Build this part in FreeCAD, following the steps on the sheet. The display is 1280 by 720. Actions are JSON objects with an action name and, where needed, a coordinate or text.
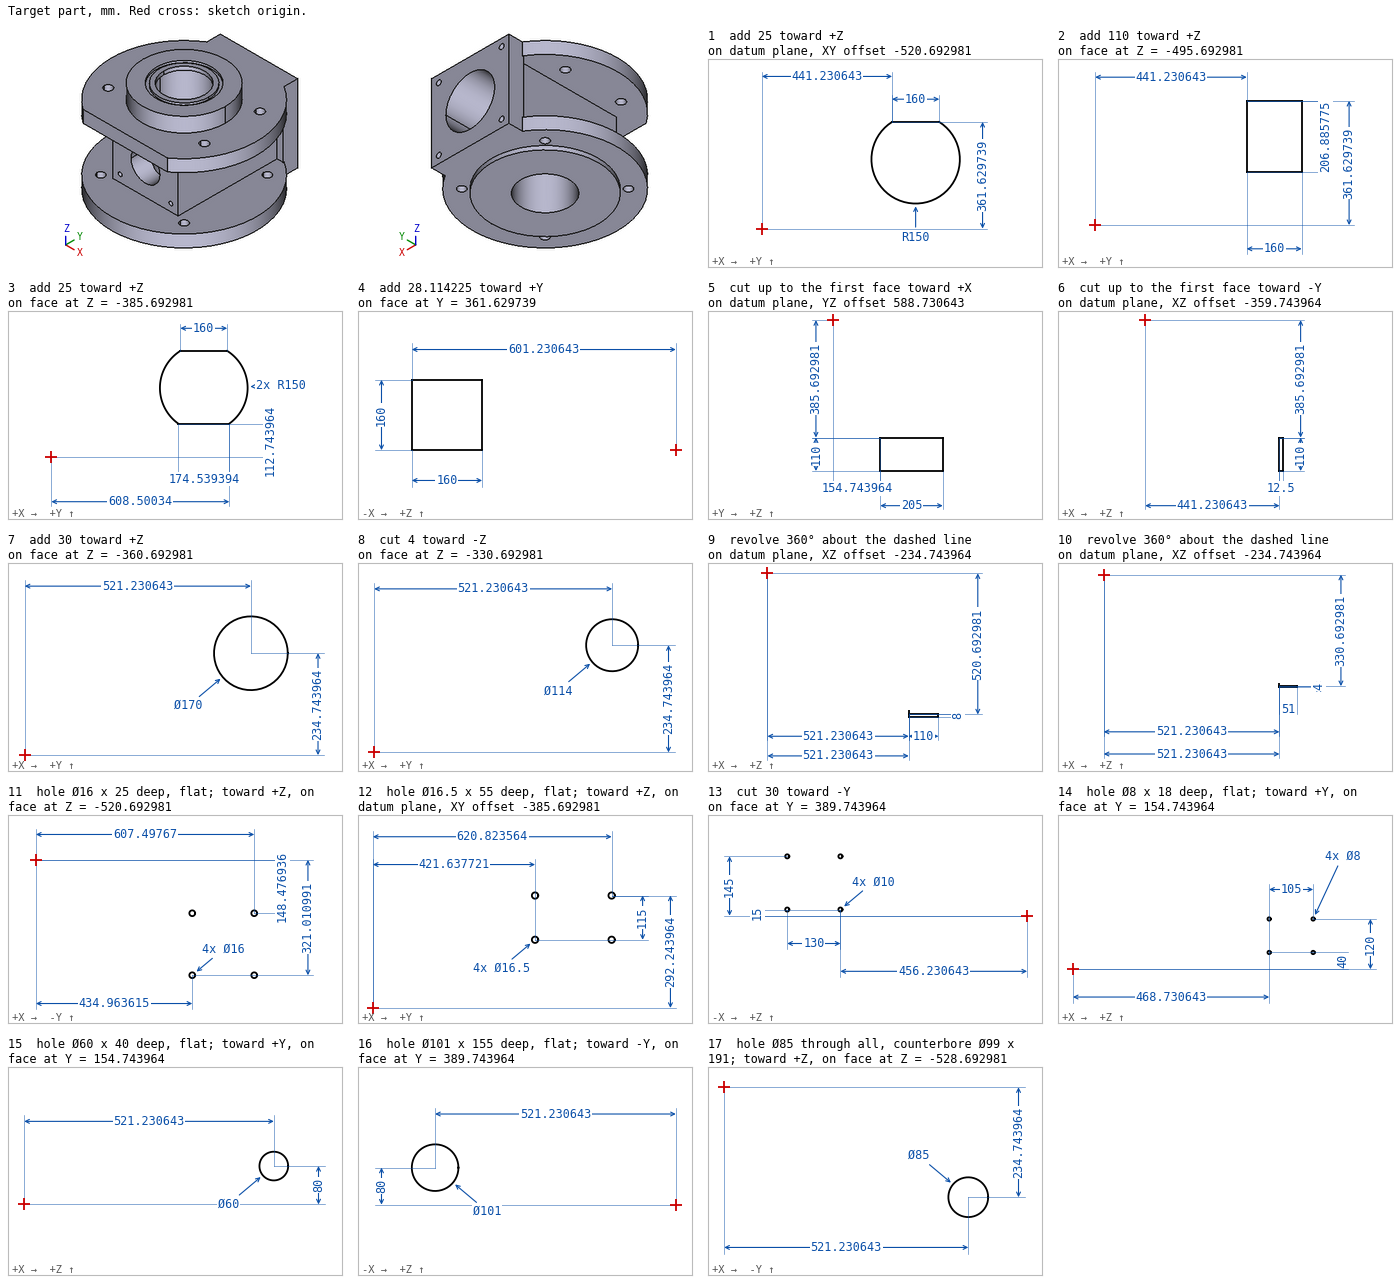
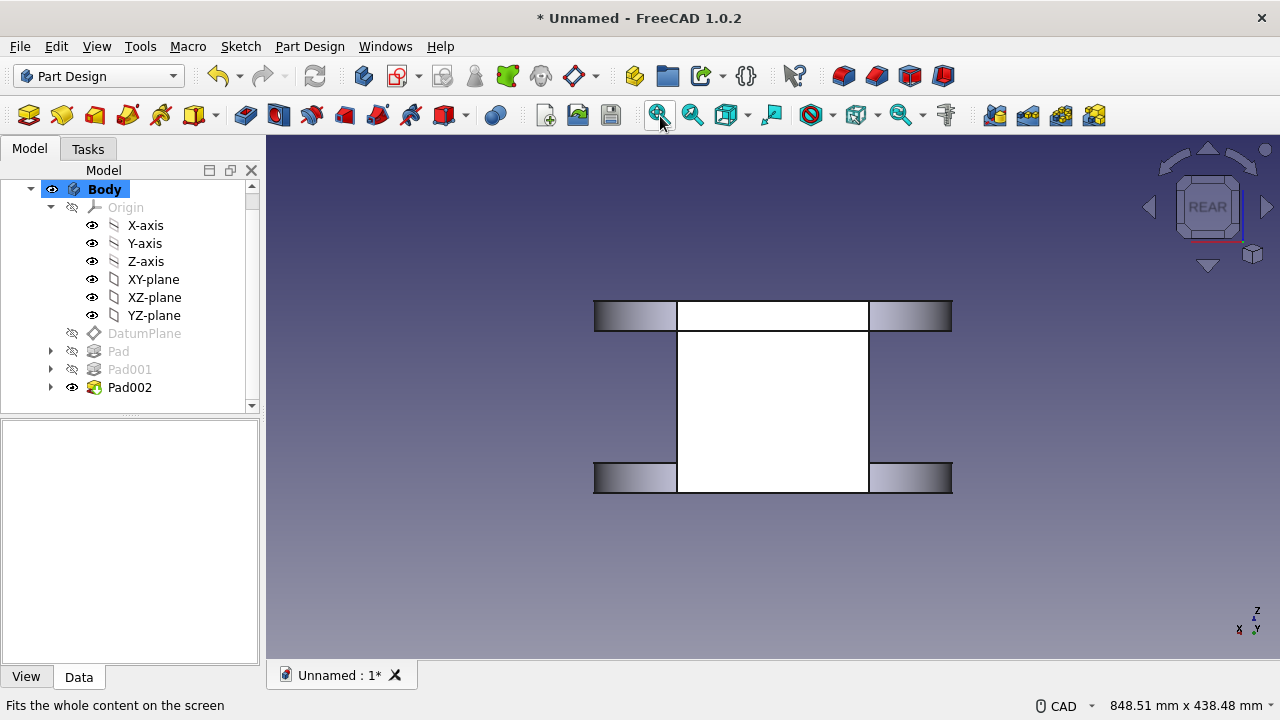
{"action": "left_click", "coordinate": [773, 411]}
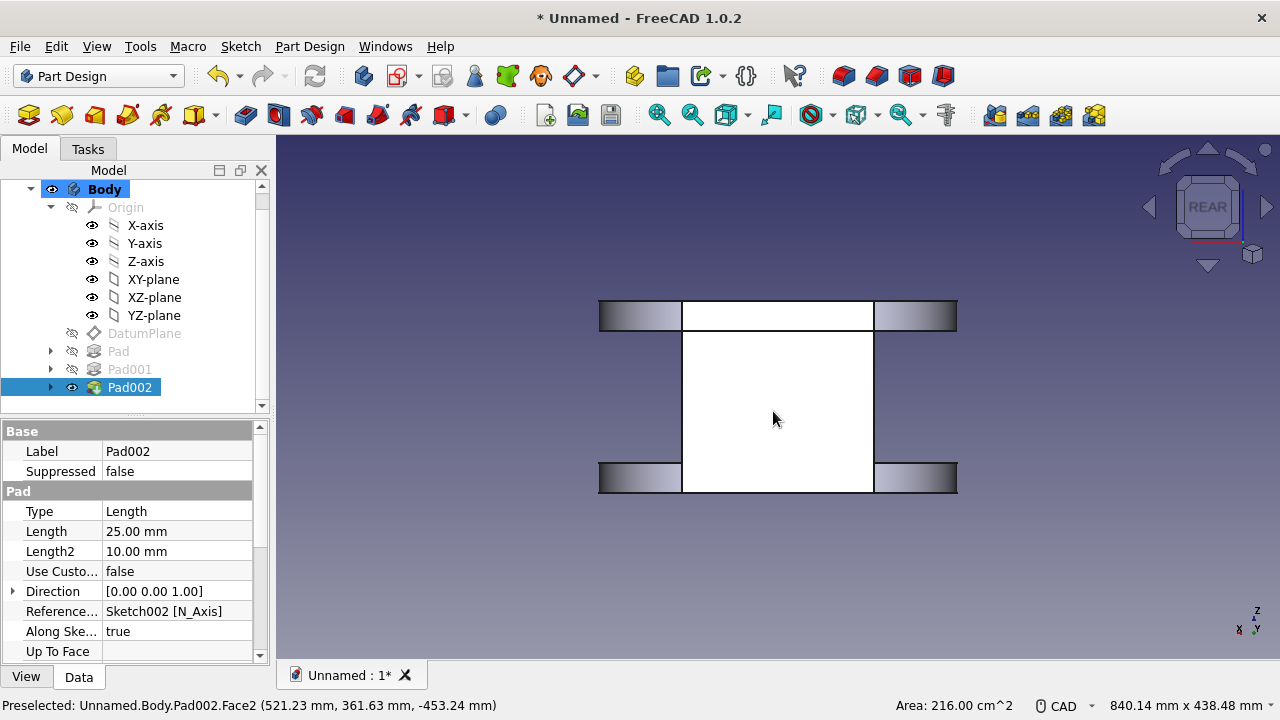
{"action": "left_click", "coordinate": [396, 76]}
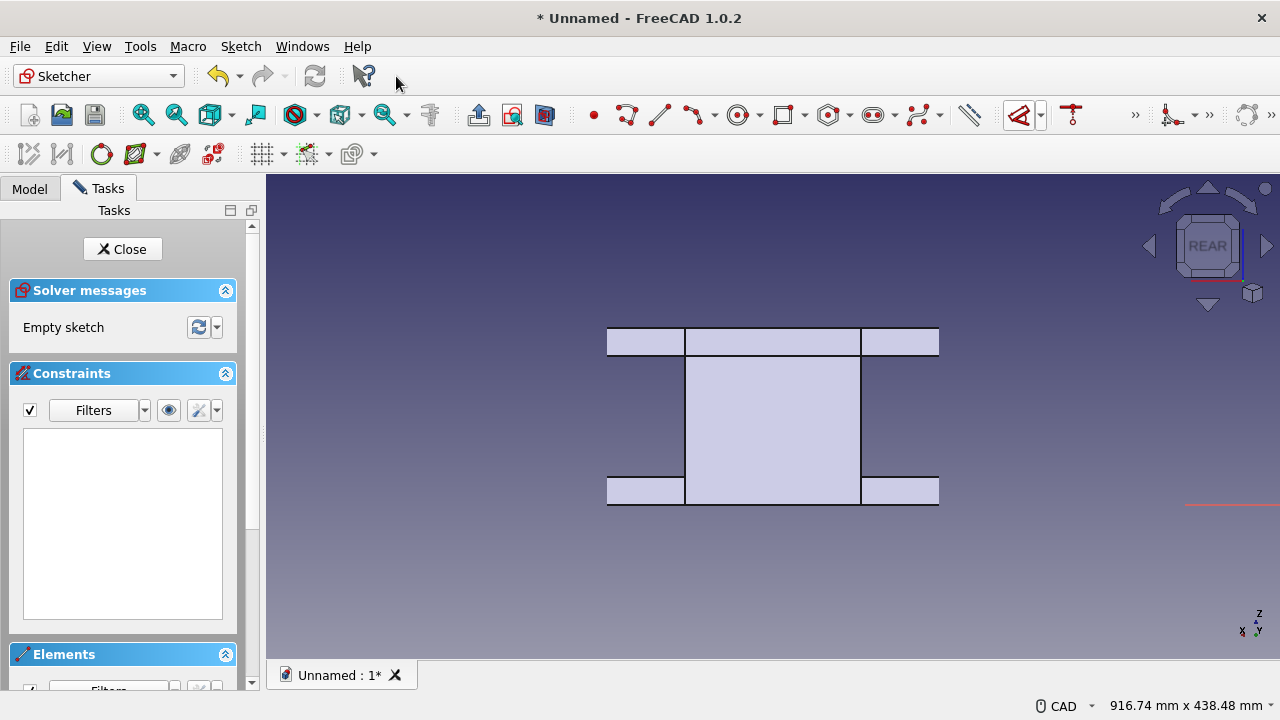
{"action": "scroll", "coordinate": [856, 416], "scroll_direction": "up", "scroll_amount": 3}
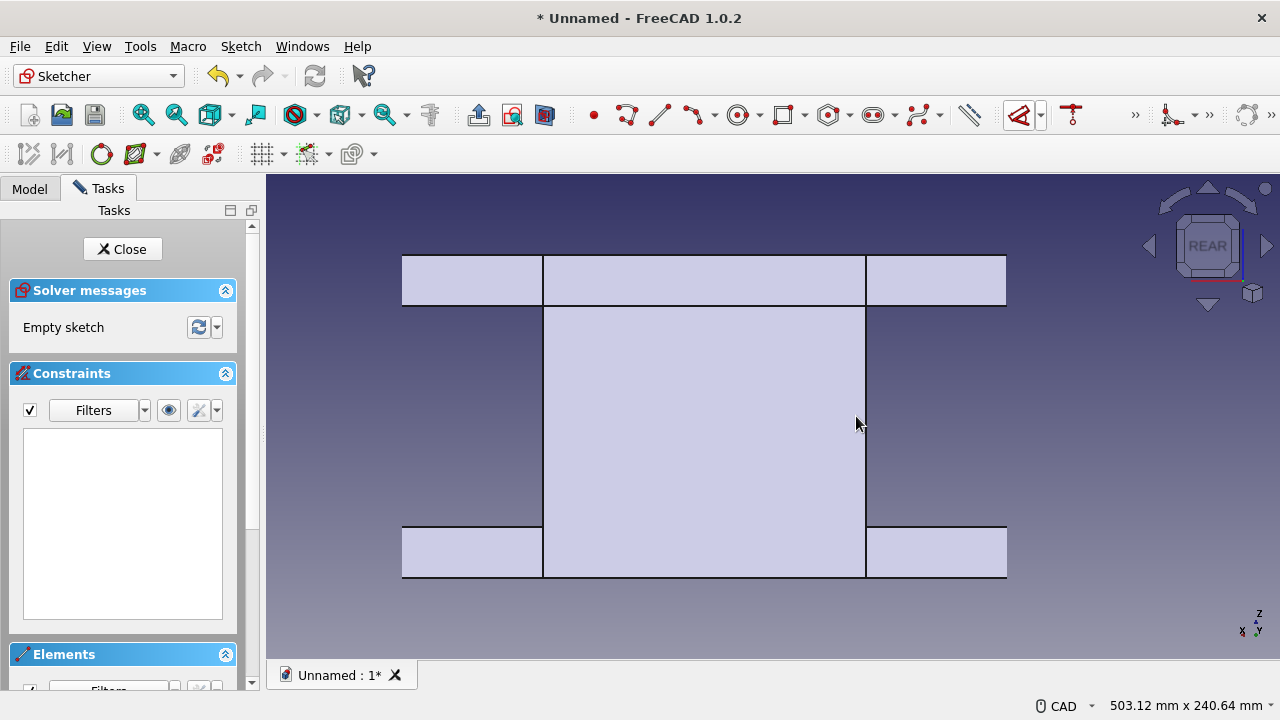
{"action": "left_click", "coordinate": [782, 116]}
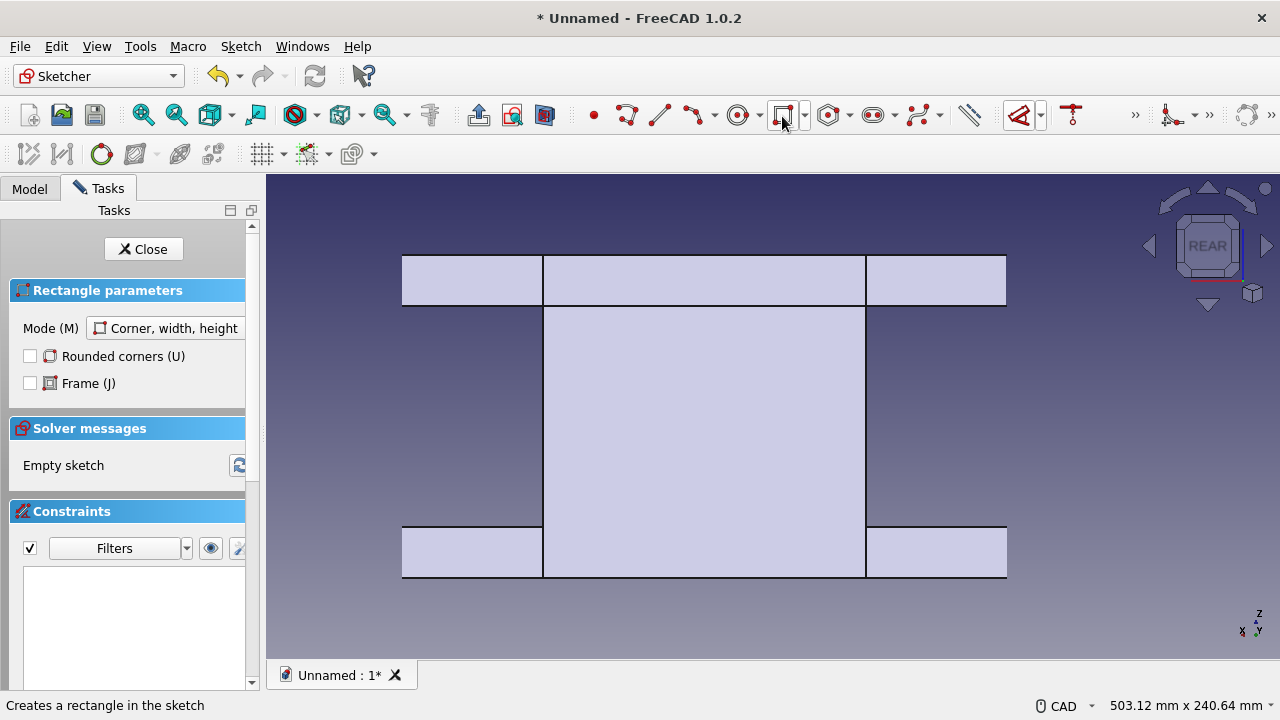
{"action": "left_click", "coordinate": [543, 255]}
{"action": "left_click", "coordinate": [866, 578]}
{"action": "key", "text": "Escape"}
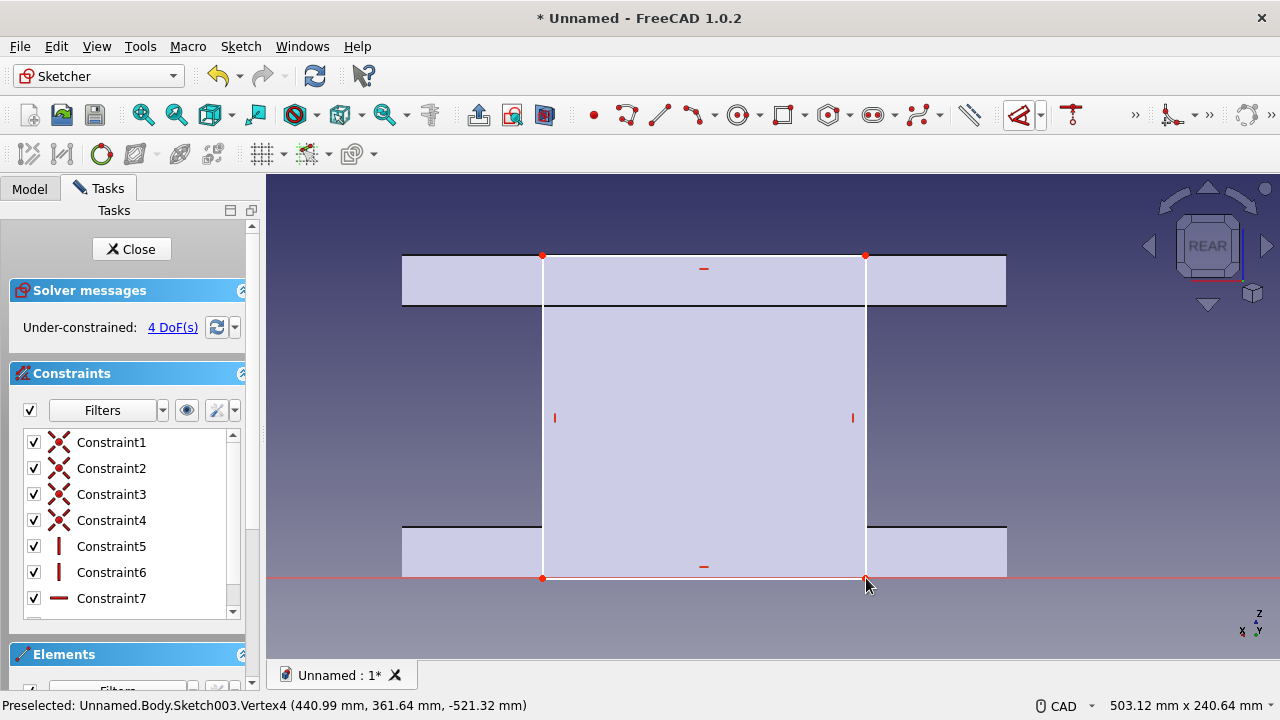
{"action": "left_click", "coordinate": [543, 579]}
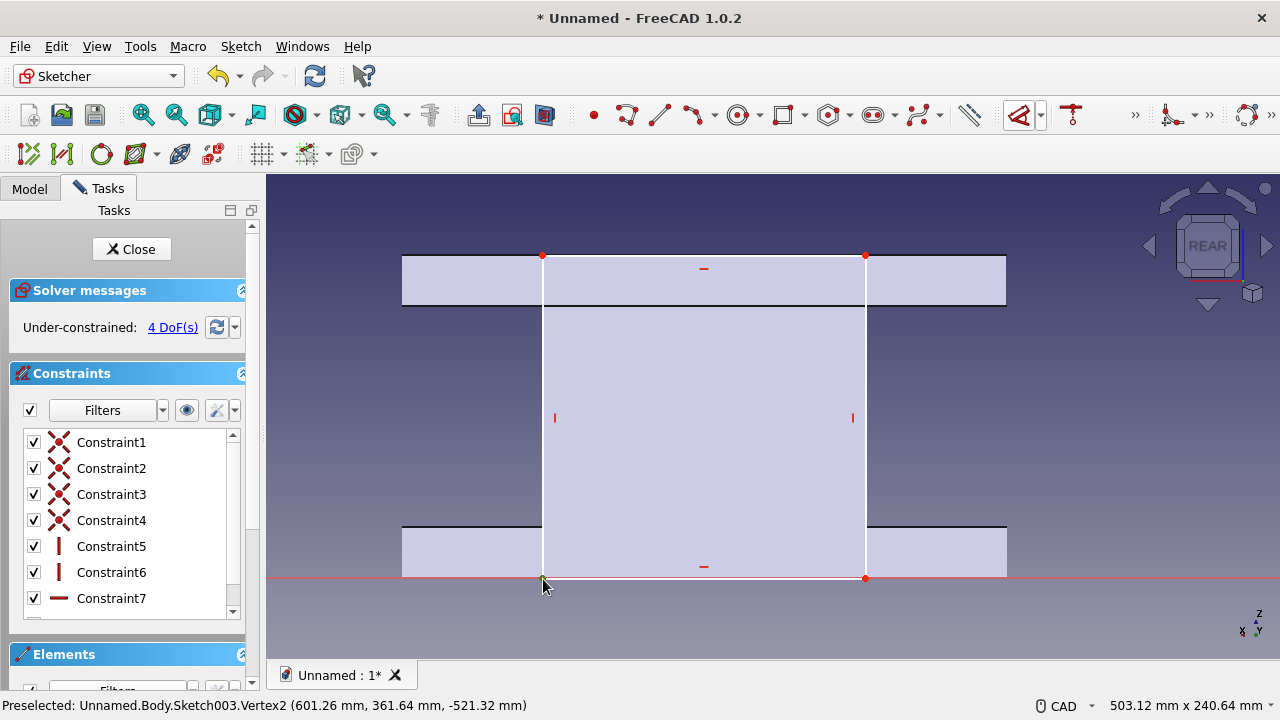
{"action": "left_click", "coordinate": [353, 578]}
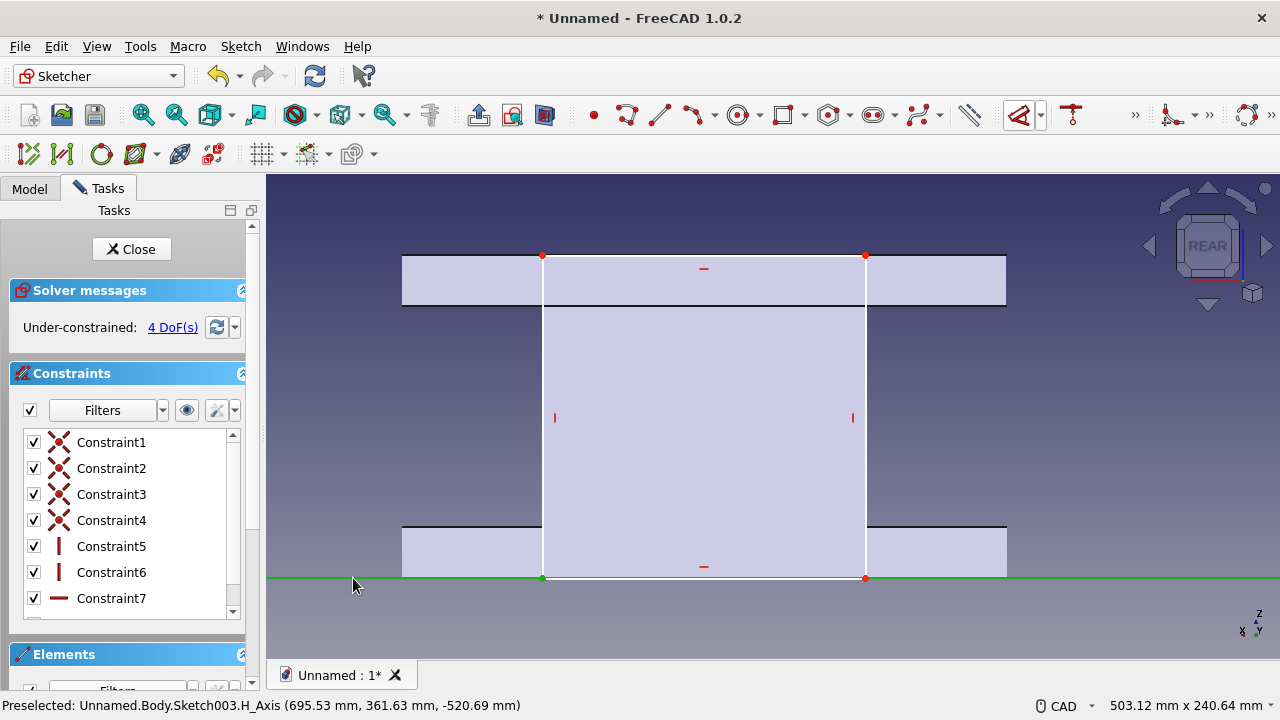
{"action": "left_click", "coordinate": [1071, 116]}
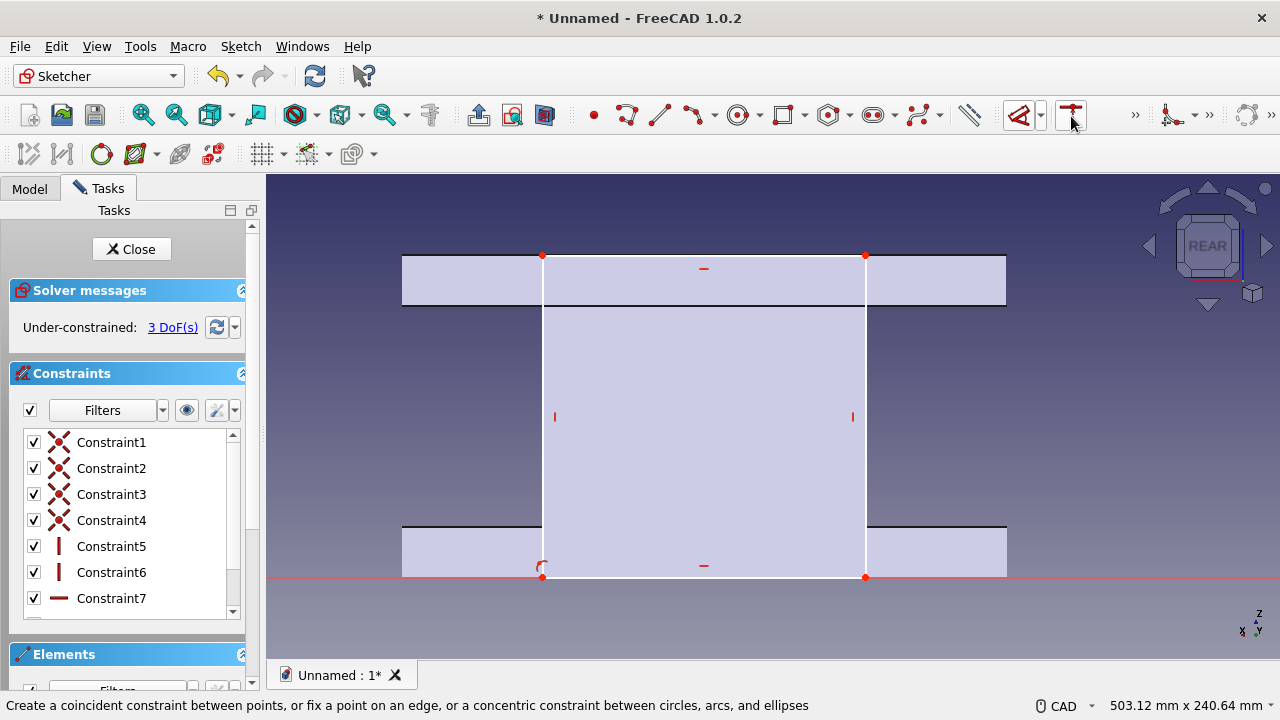
{"action": "left_click", "coordinate": [543, 353]}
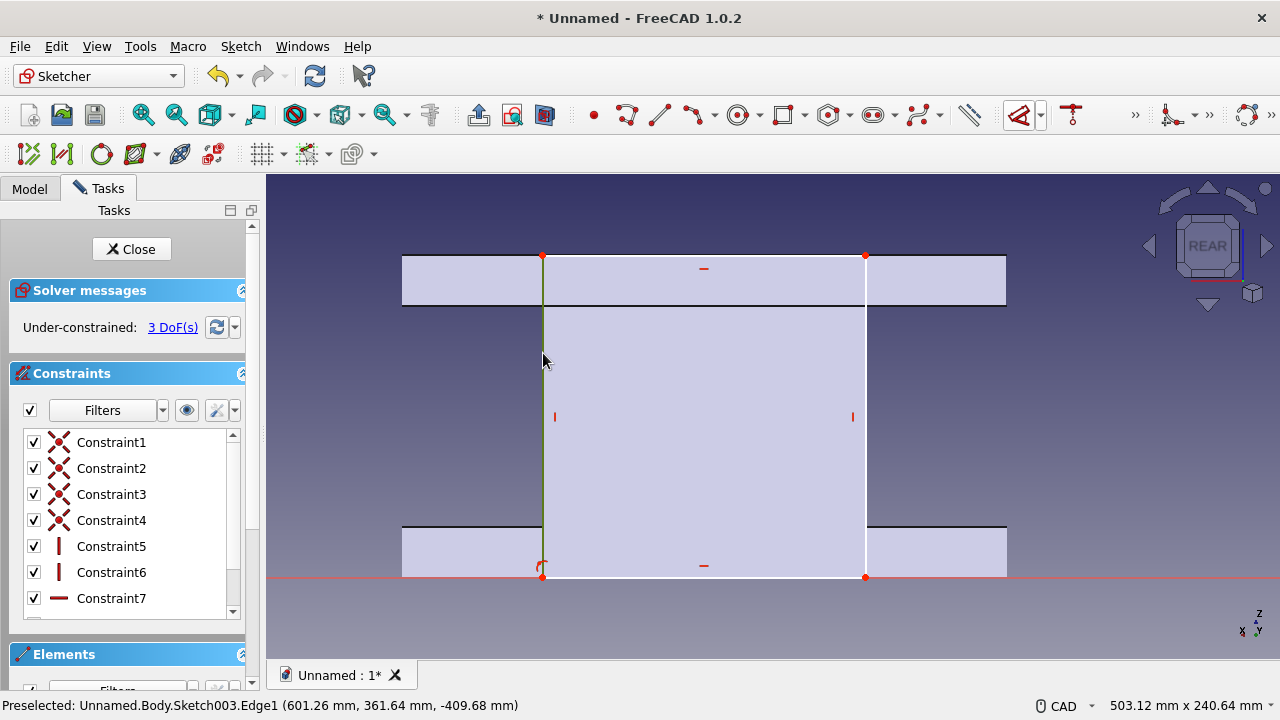
{"action": "left_click", "coordinate": [1040, 116]}